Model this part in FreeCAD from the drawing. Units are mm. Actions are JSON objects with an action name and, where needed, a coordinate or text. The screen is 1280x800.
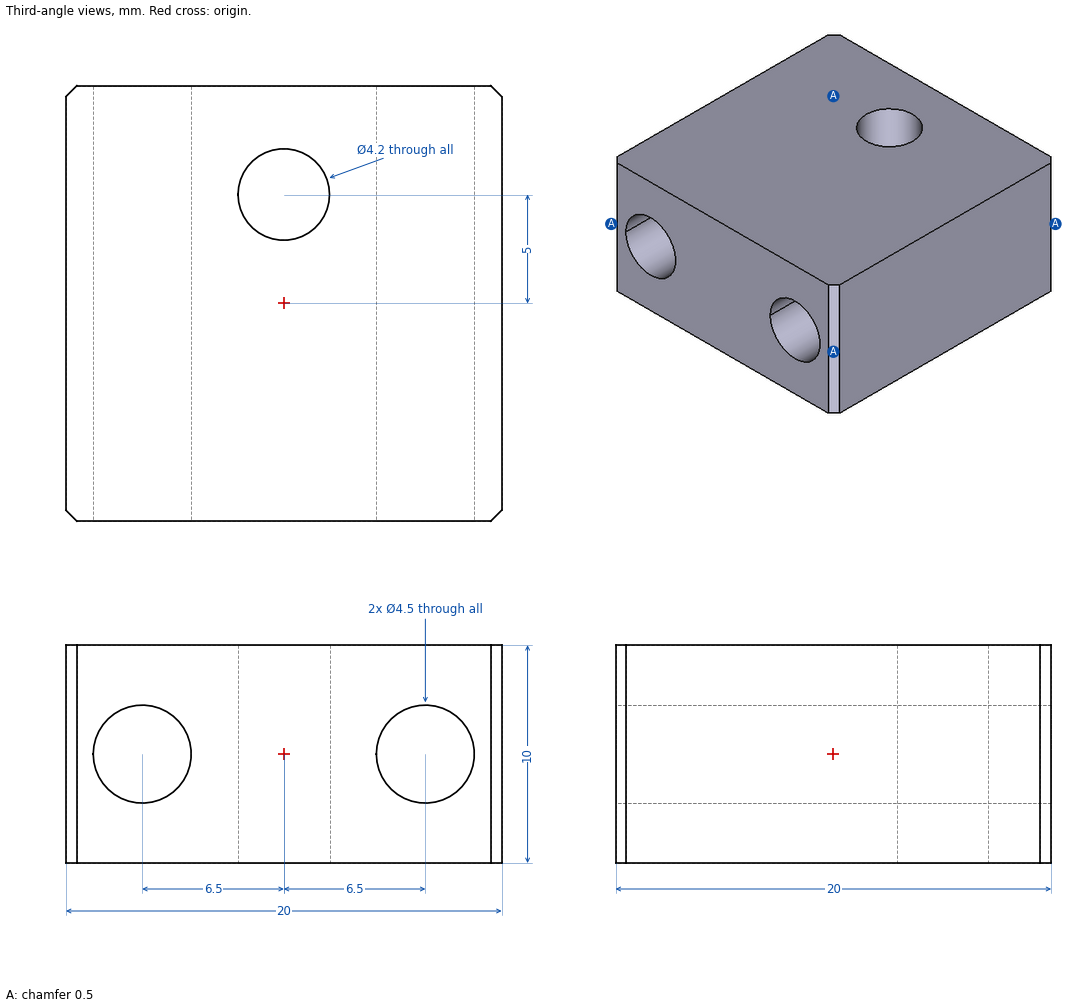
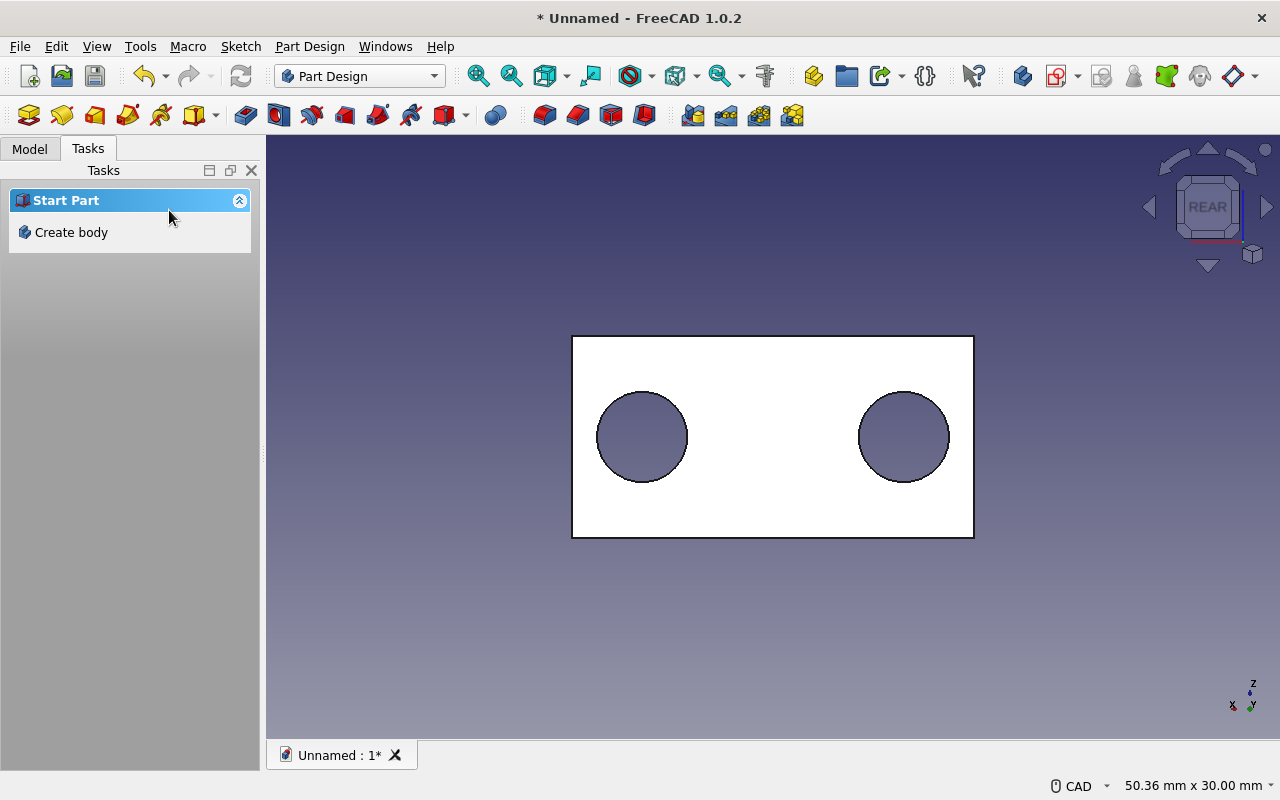
{"action": "left_click", "coordinate": [479, 76]}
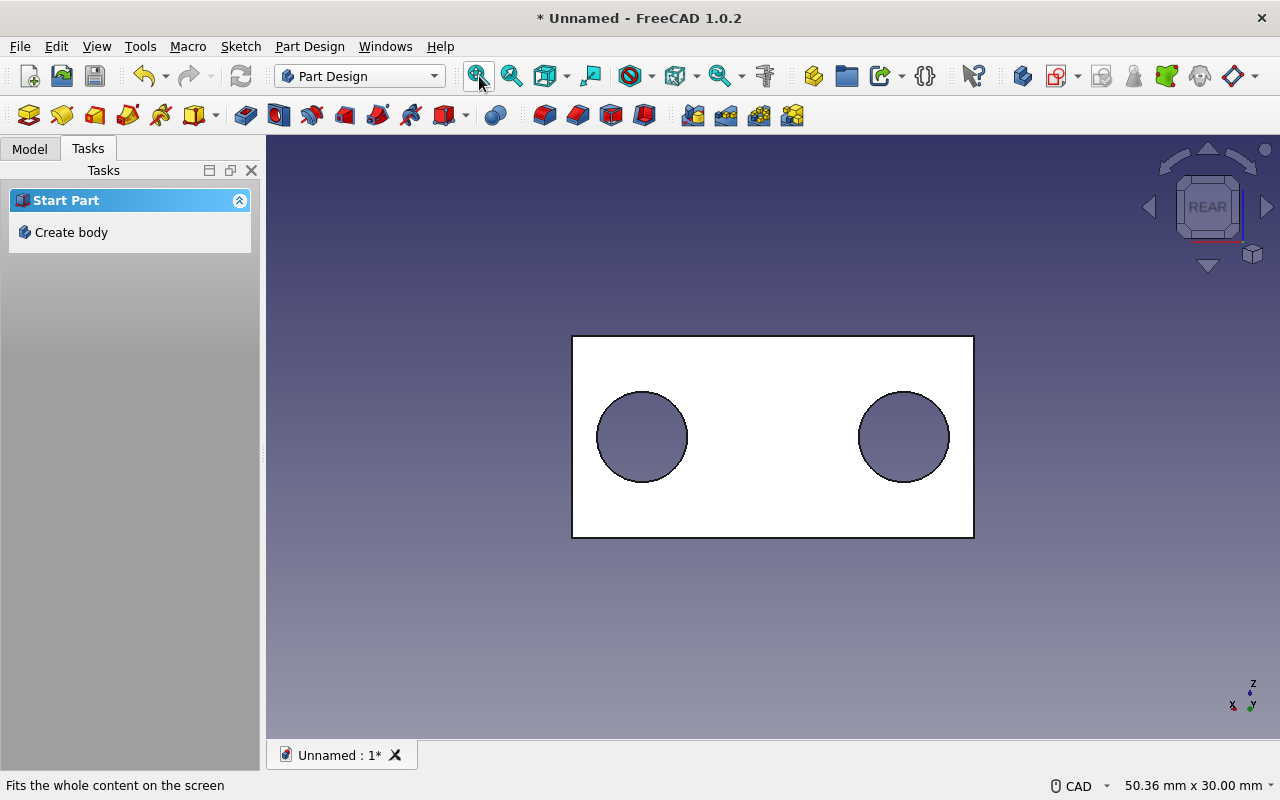
{"action": "left_click", "coordinate": [974, 436]}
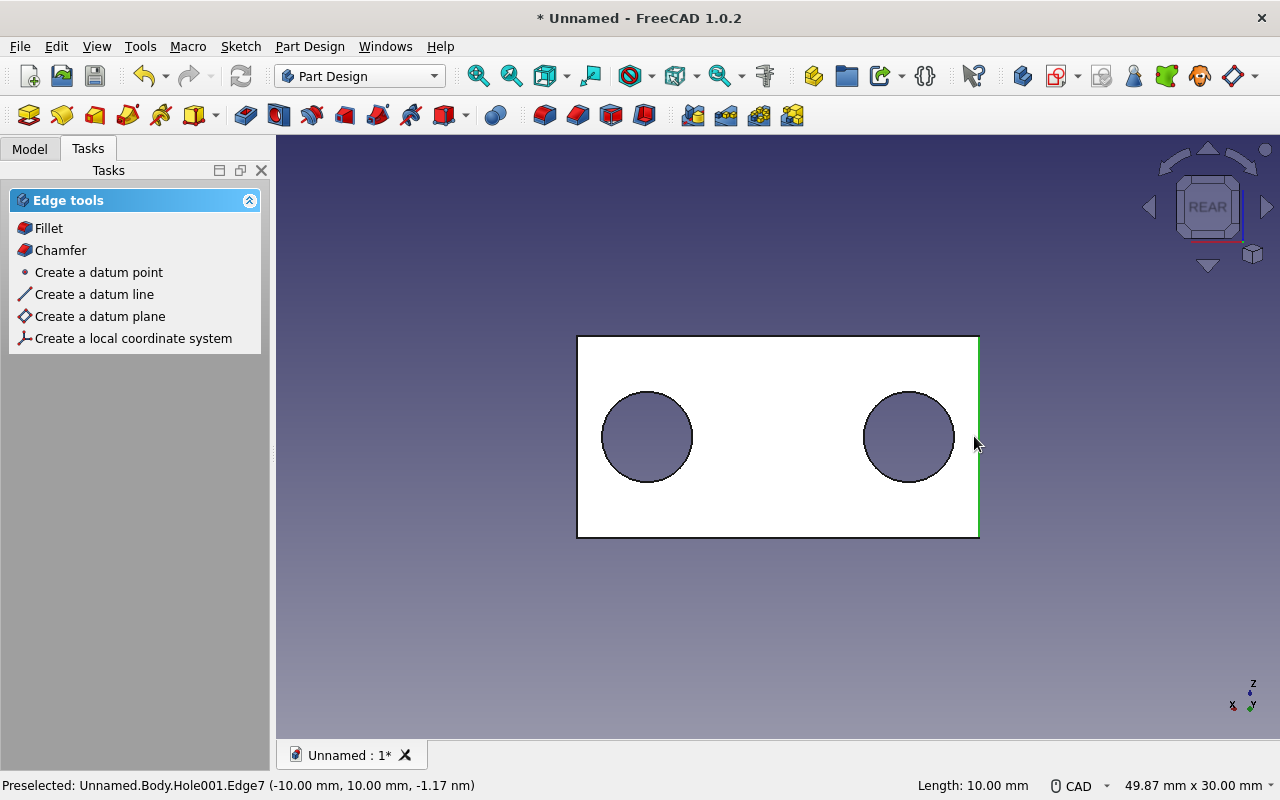
{"action": "key", "text": "0"}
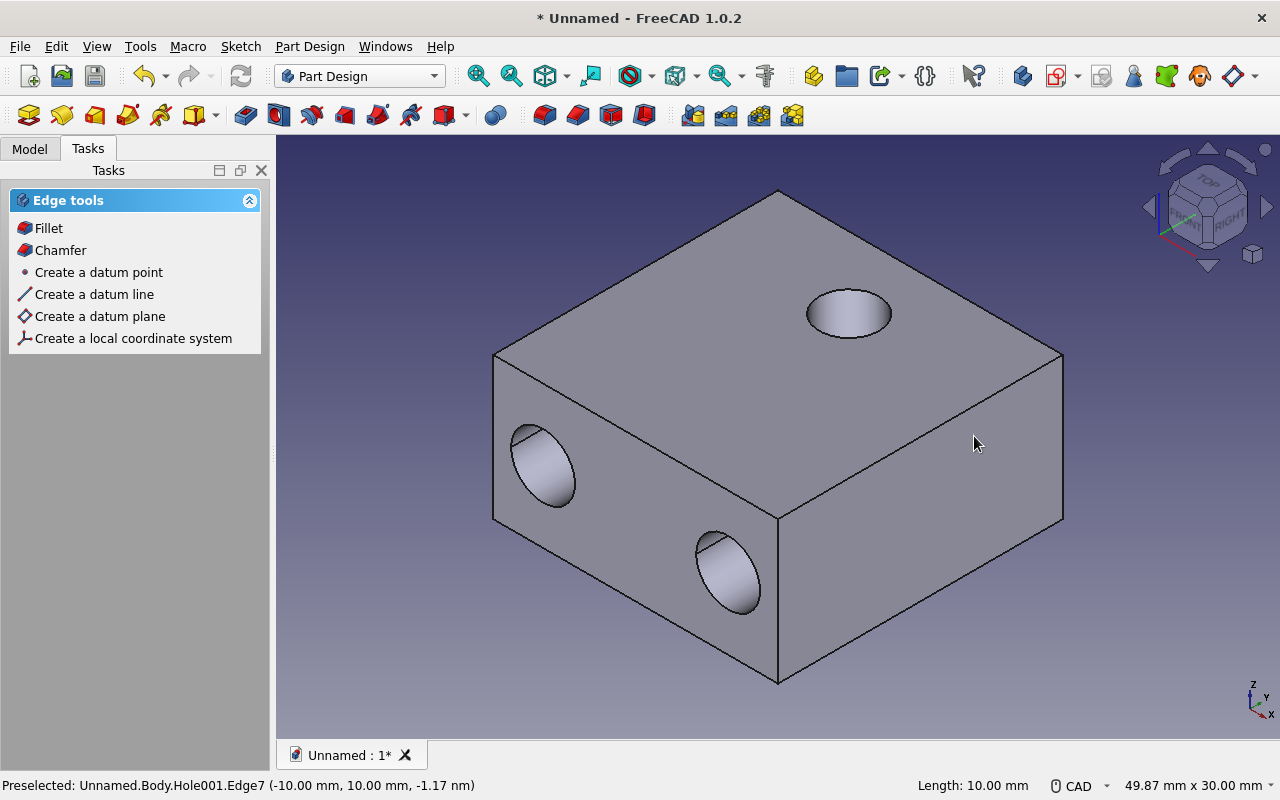
{"action": "left_click", "coordinate": [778, 600], "text": "ctrl"}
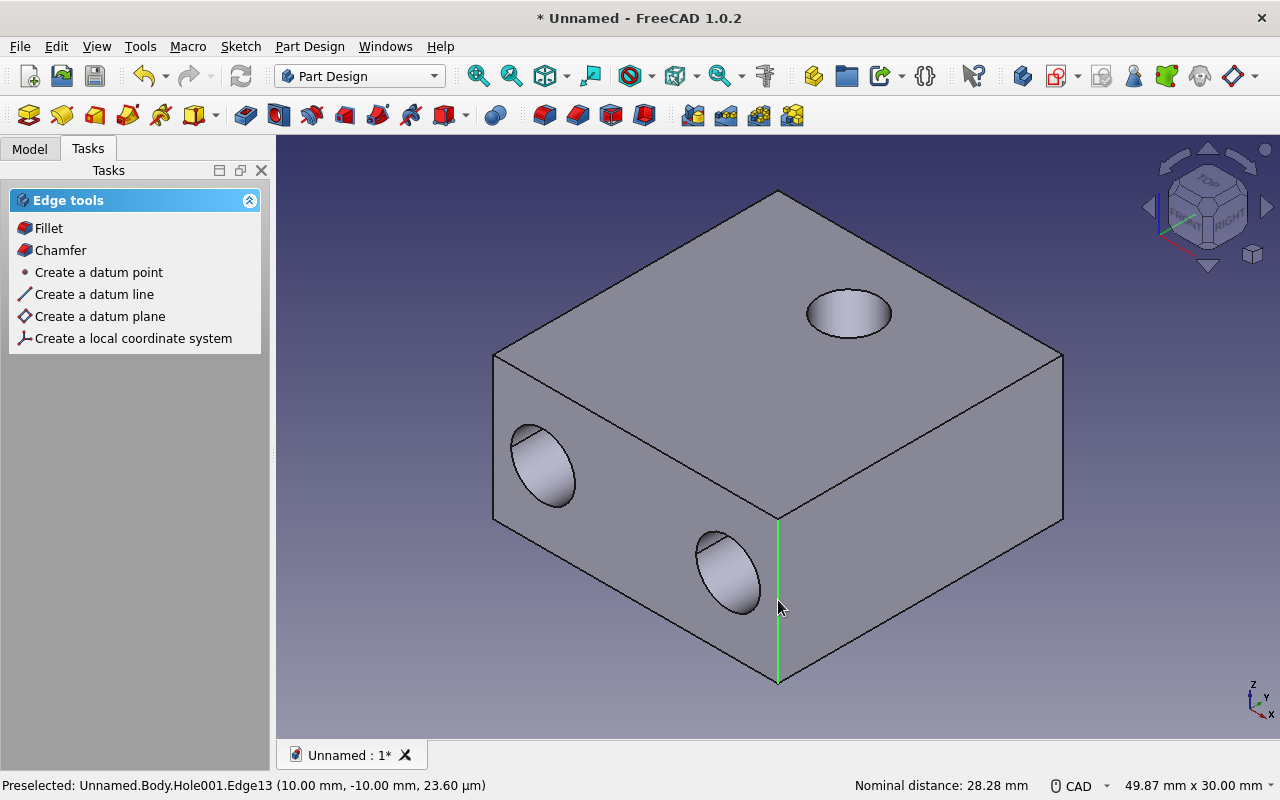
{"action": "key", "text": "2"}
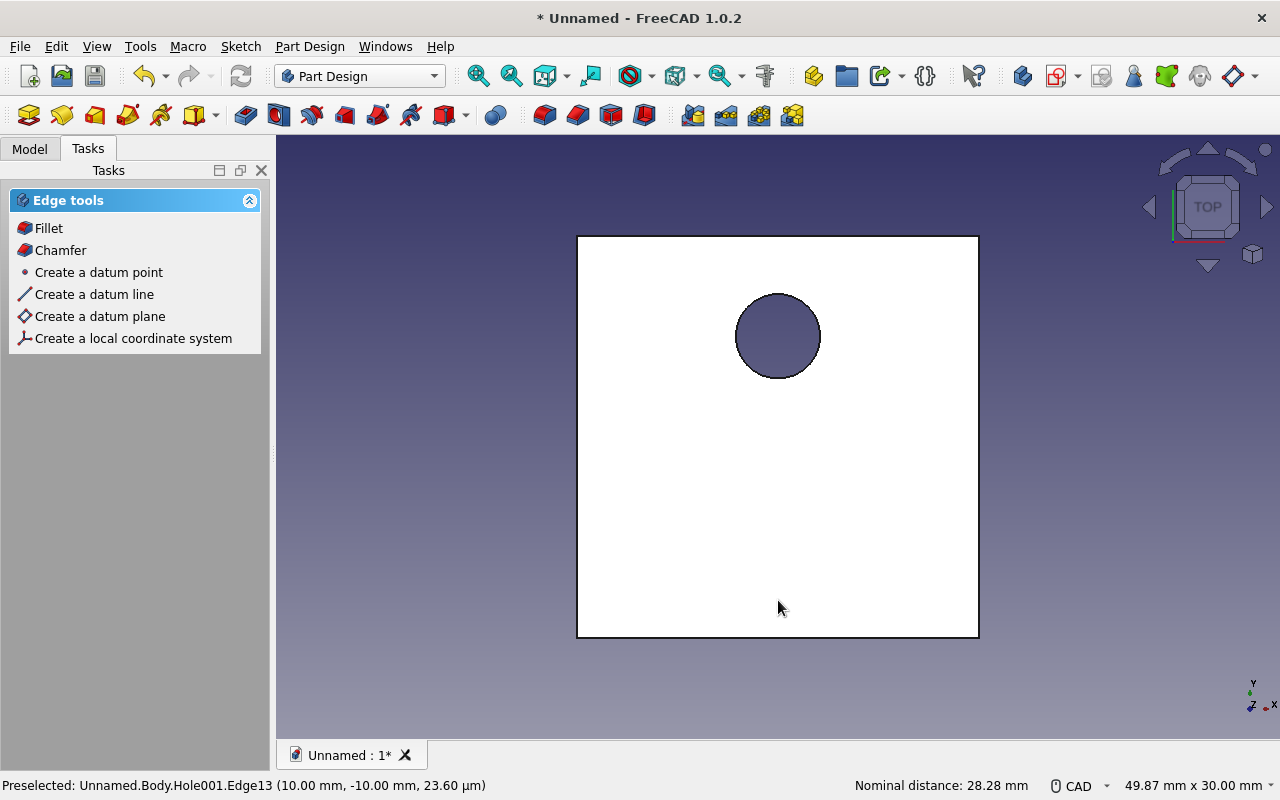
{"action": "key", "text": "1"}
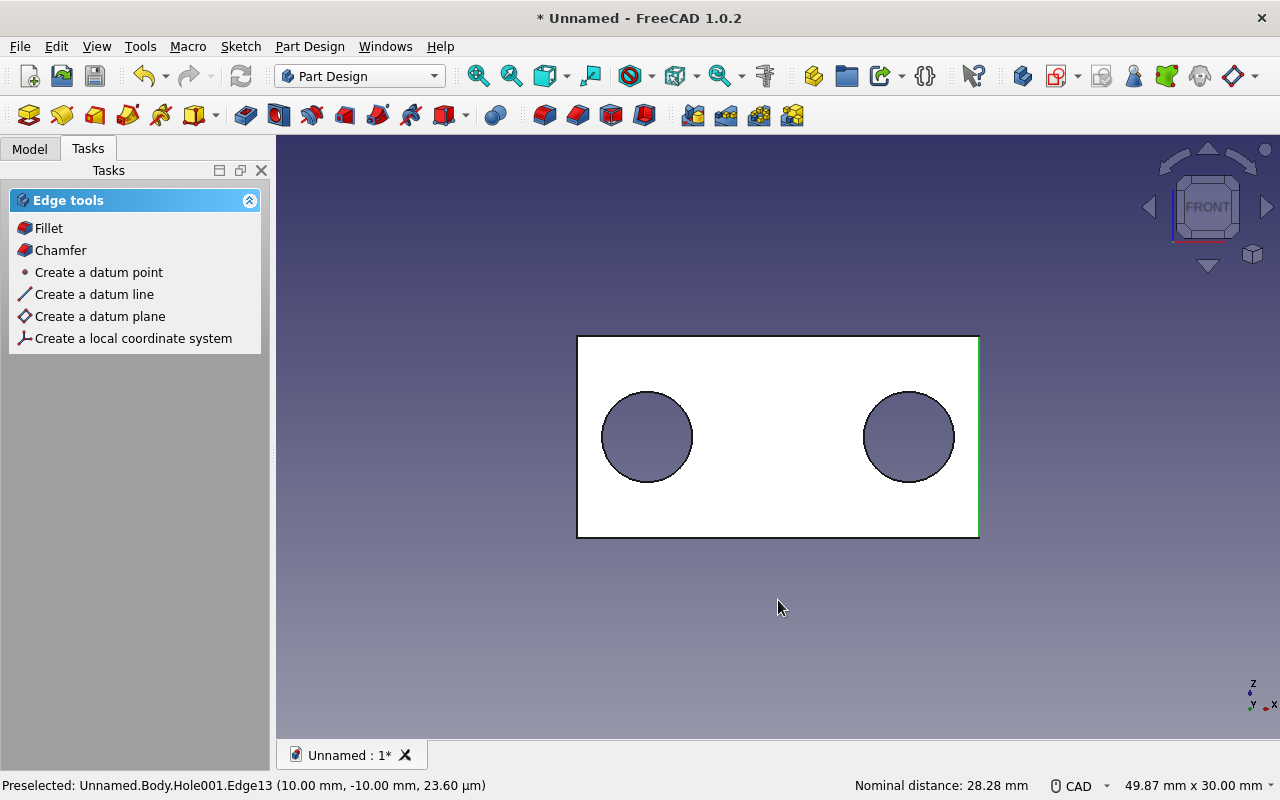
{"action": "key", "text": "v f"}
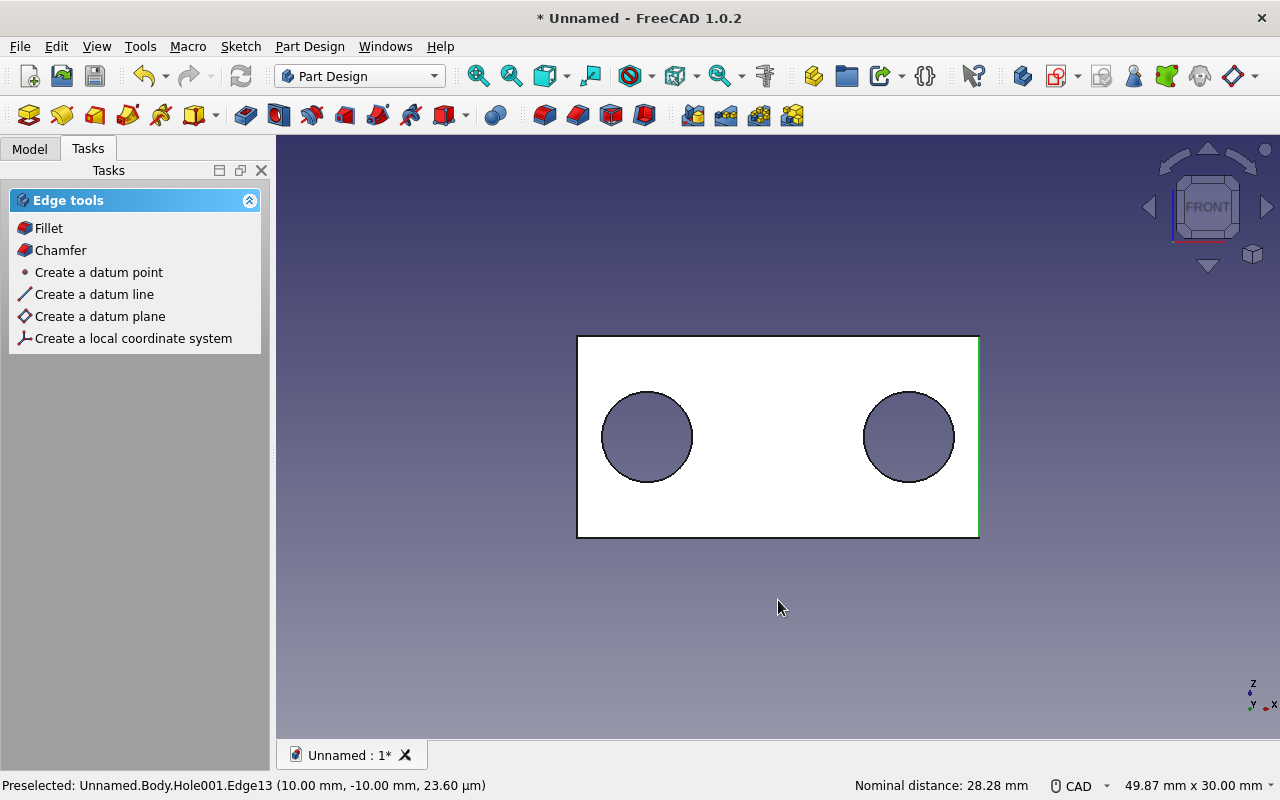
{"action": "left_click", "coordinate": [577, 436], "text": "ctrl"}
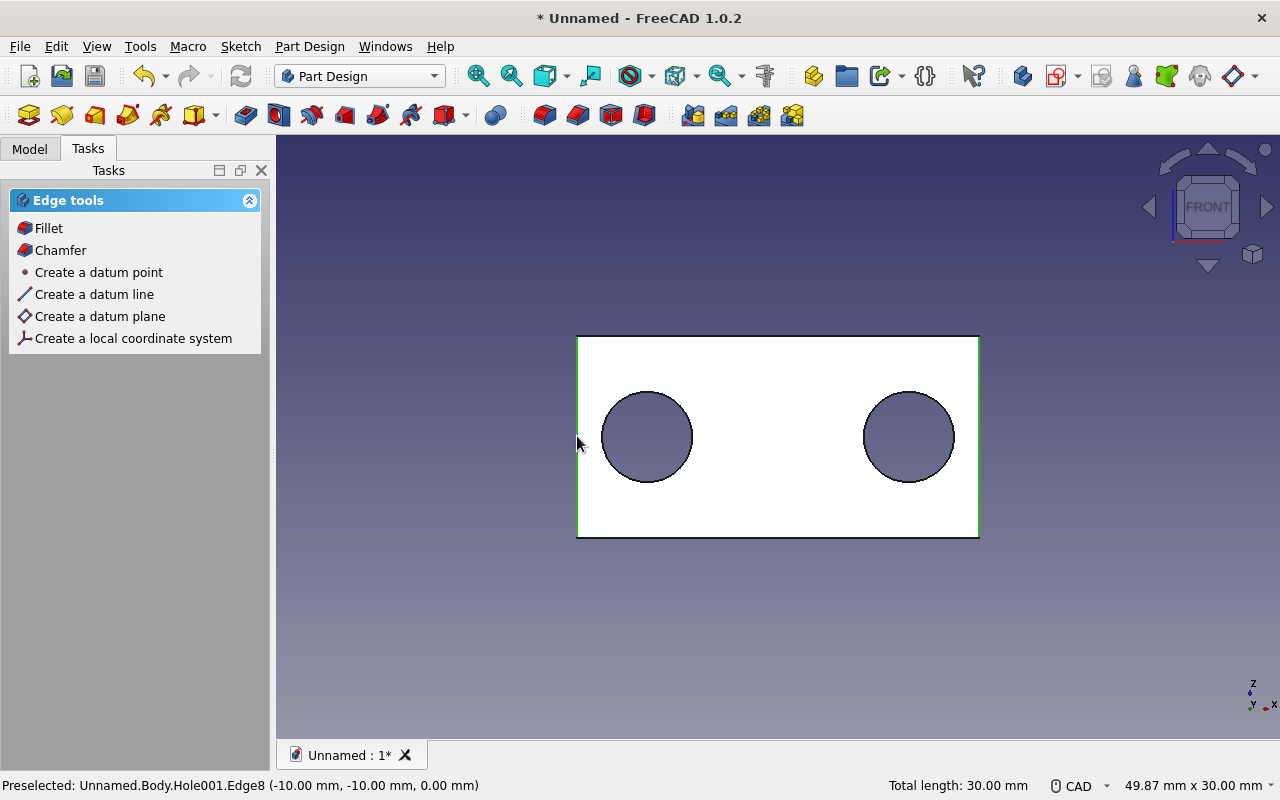
{"action": "key", "text": "3"}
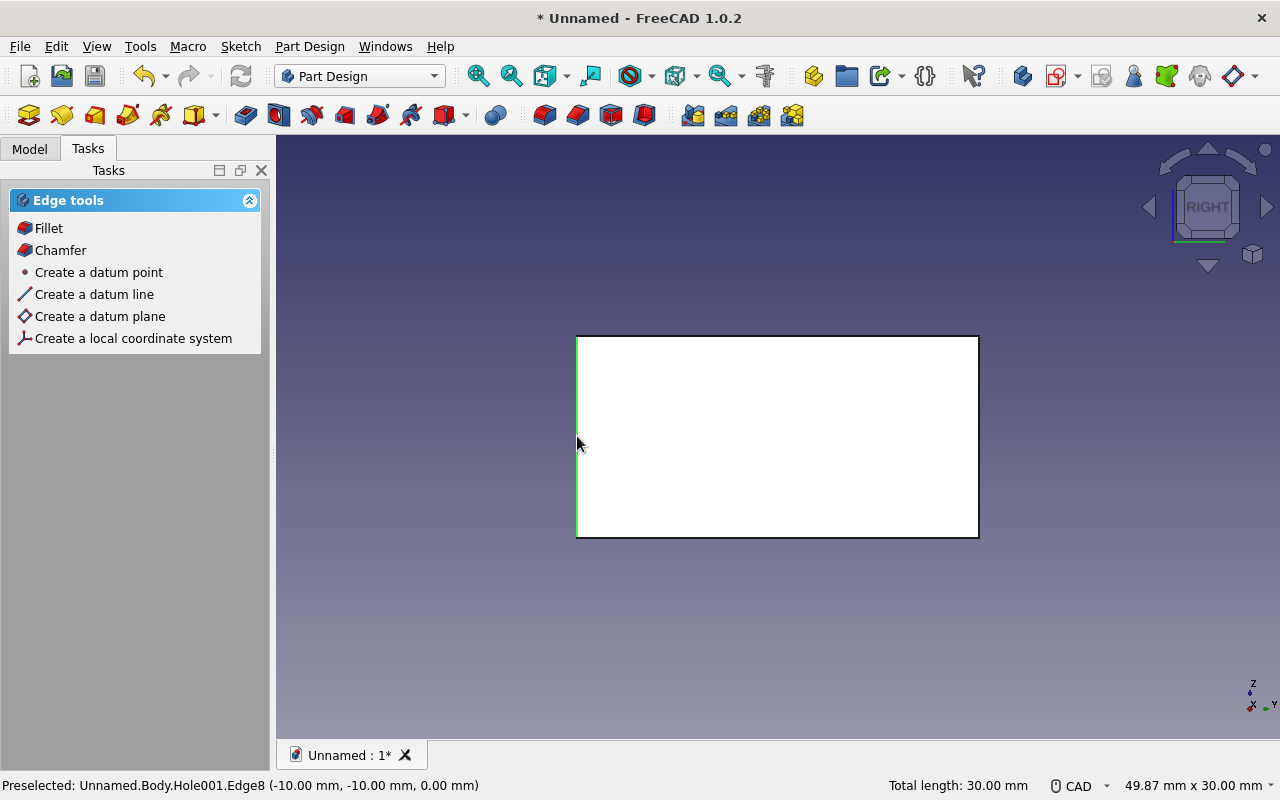
{"action": "key", "text": "v f"}